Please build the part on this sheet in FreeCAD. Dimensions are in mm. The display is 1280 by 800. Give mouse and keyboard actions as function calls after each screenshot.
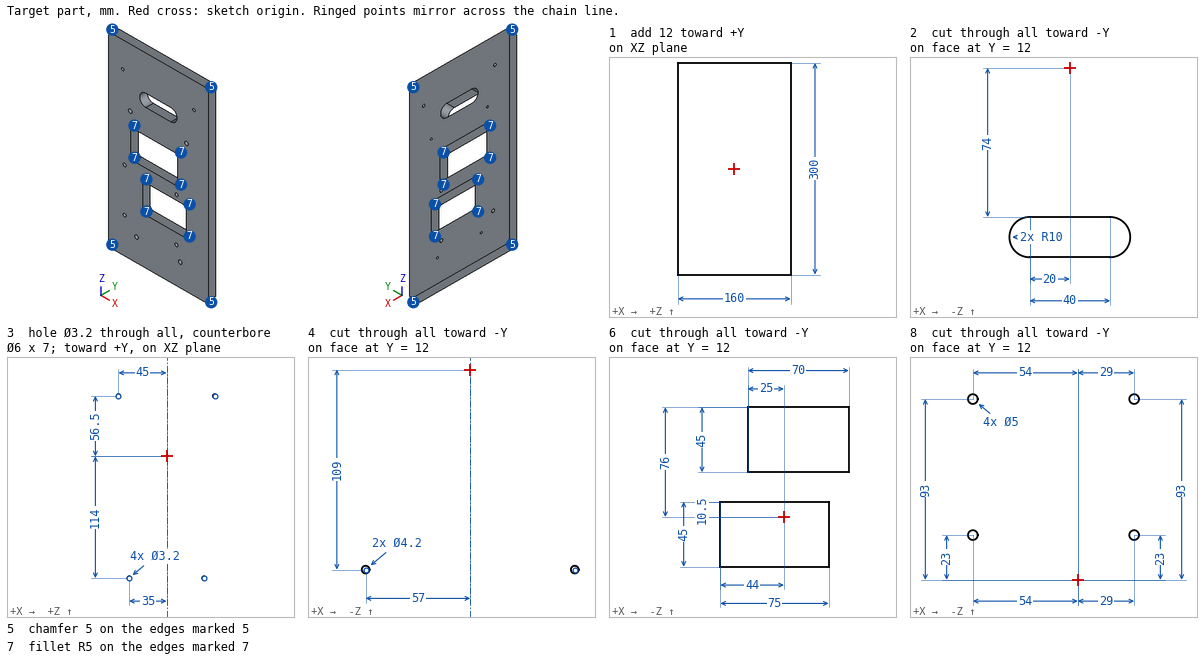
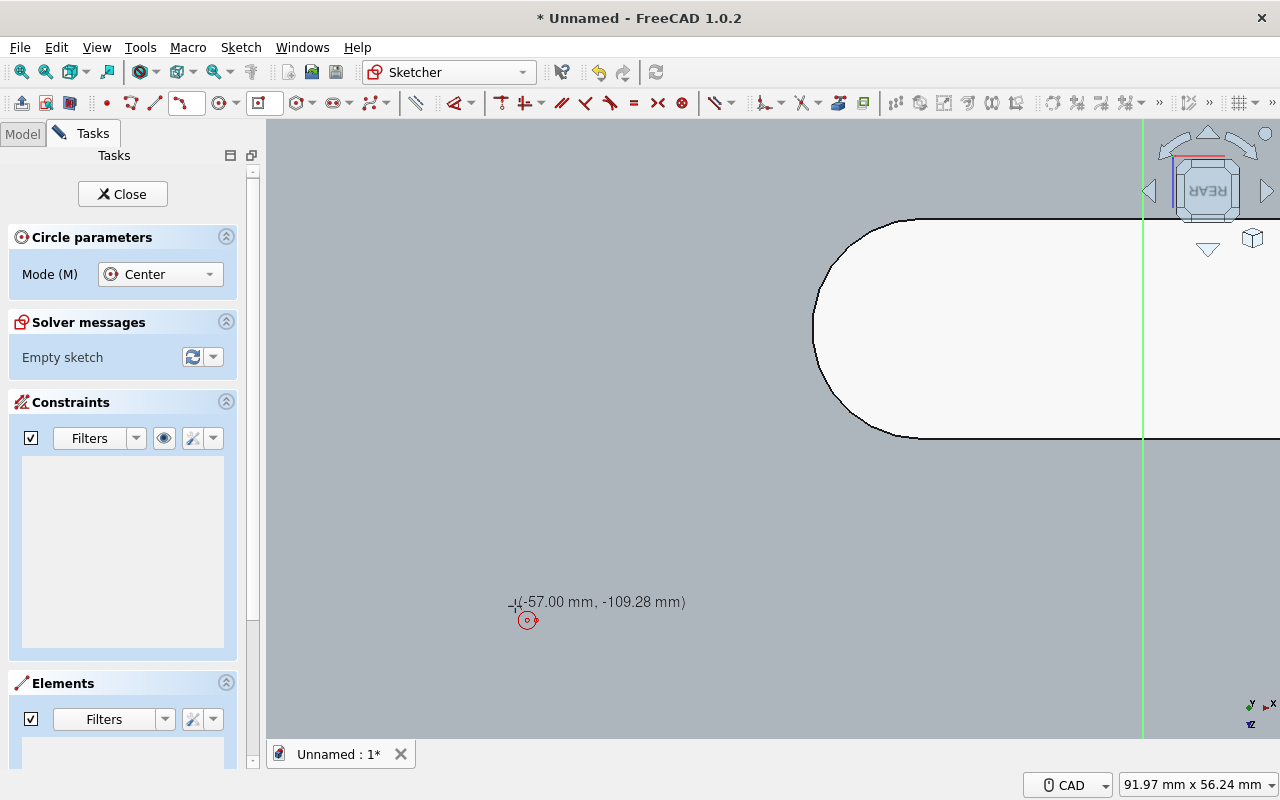
click(514, 604)
click(531, 588)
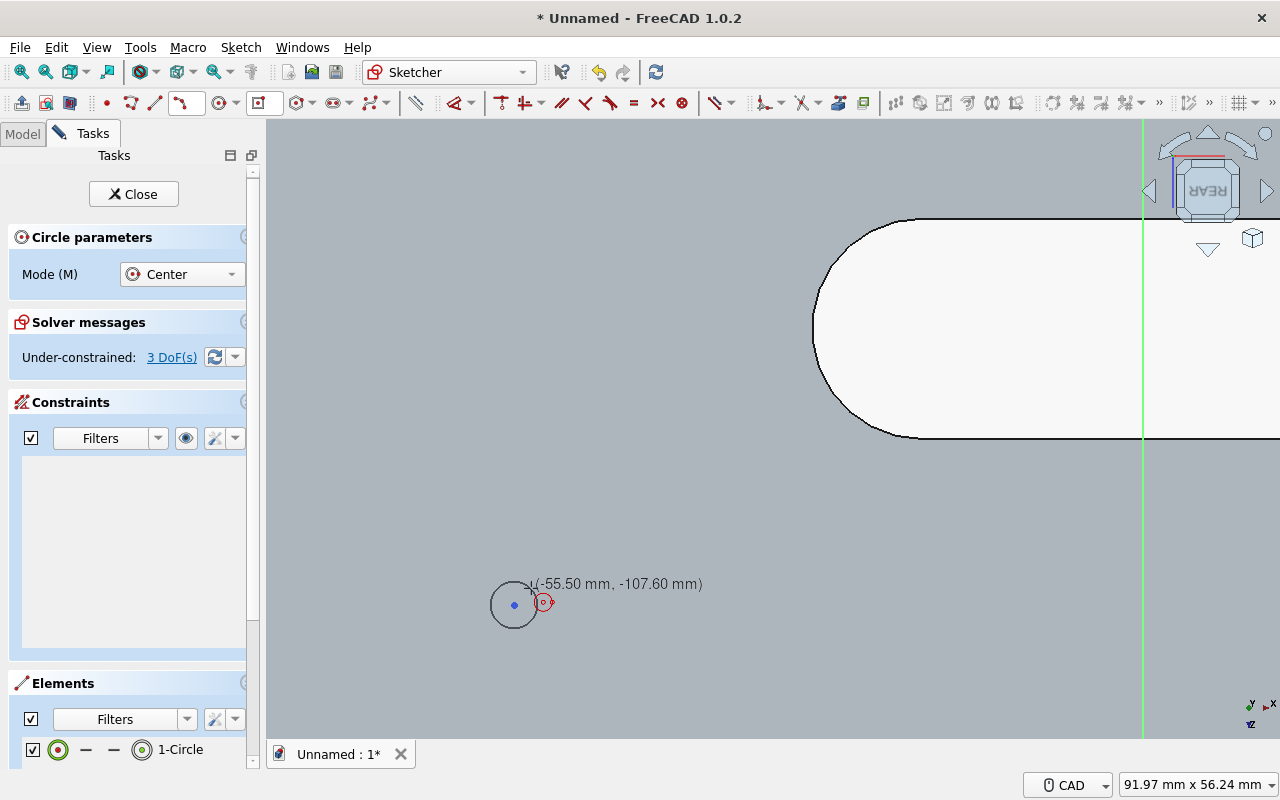
scroll(516, 607, down, 6)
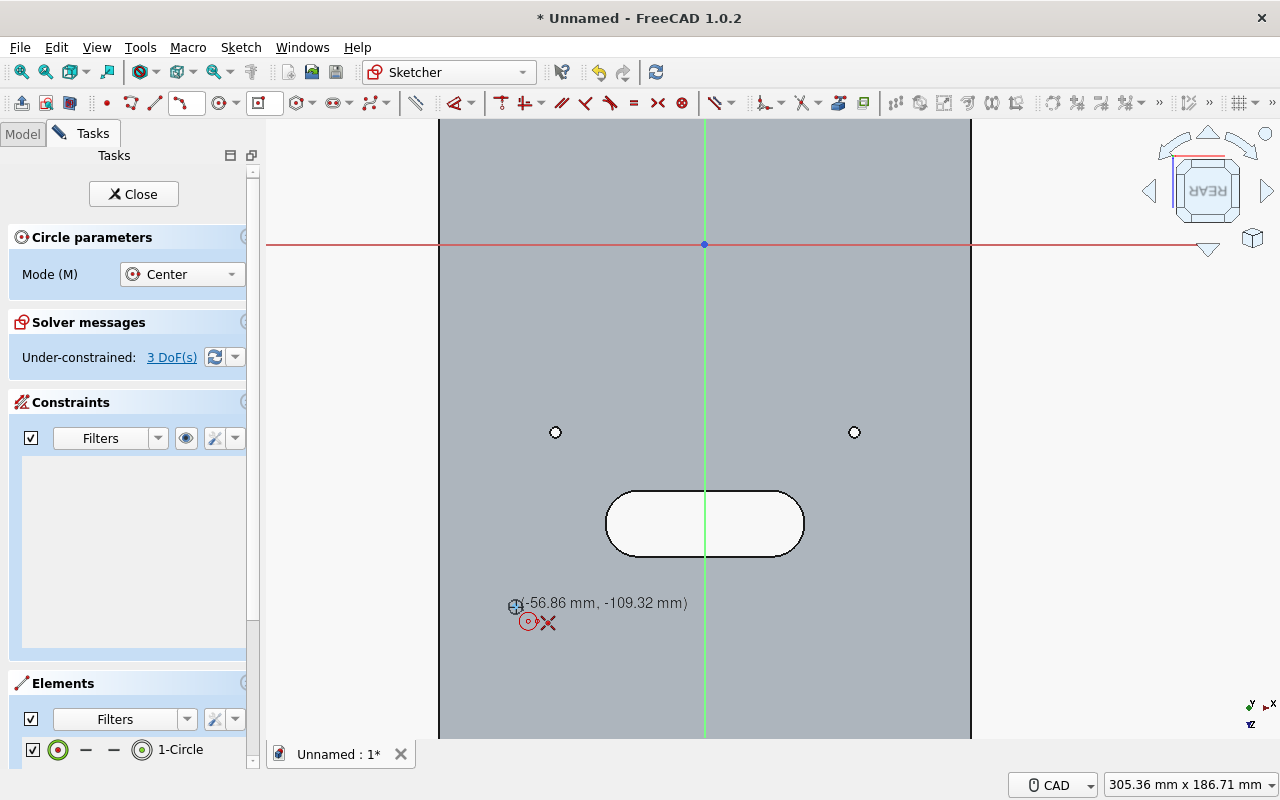
scroll(894, 607, up, 6)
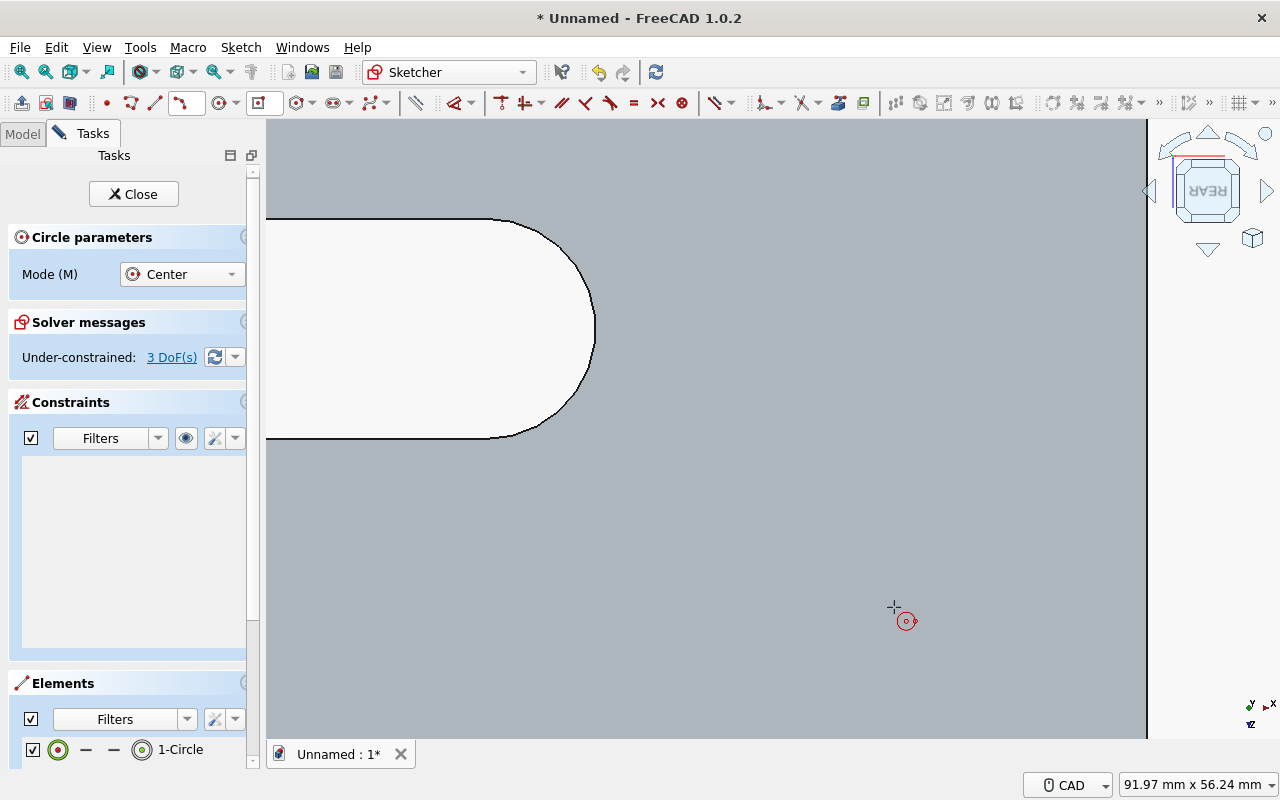
click(893, 604)
click(910, 588)
key(Escape)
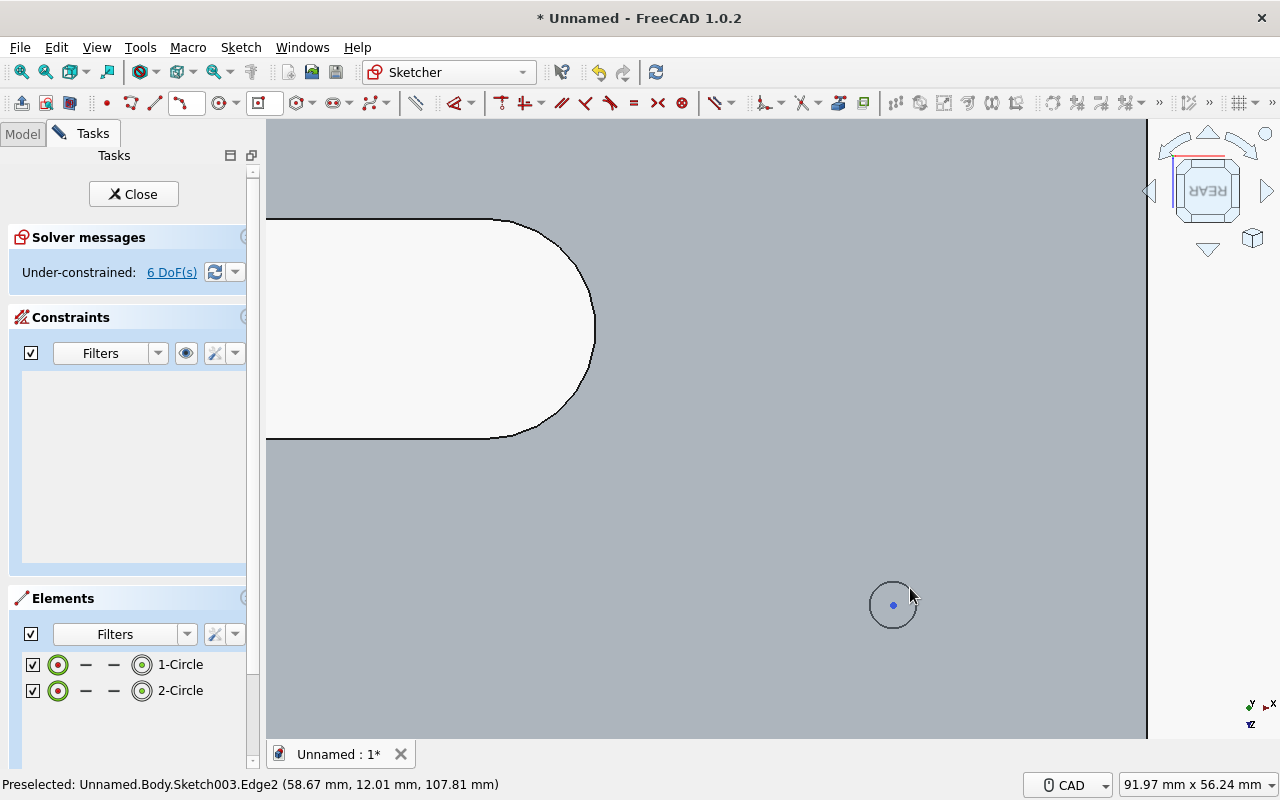
scroll(894, 607, down, 6)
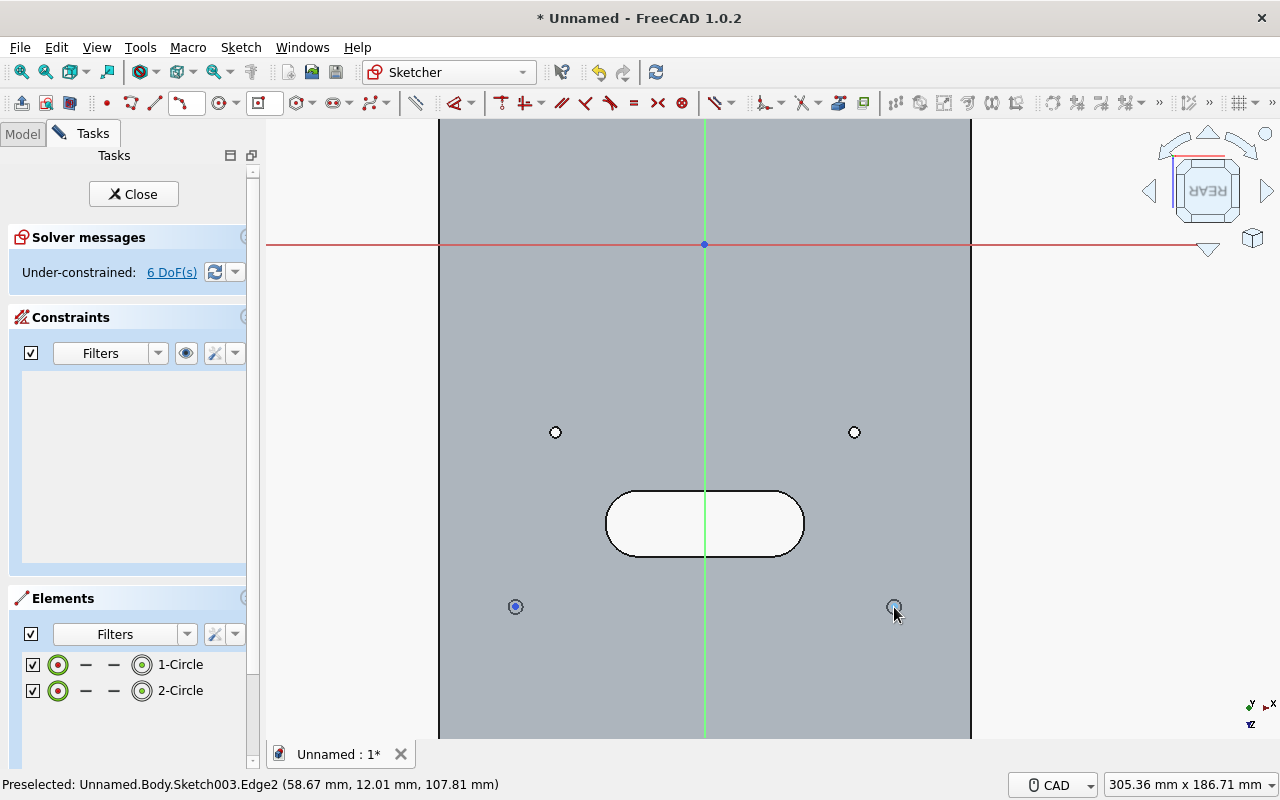
scroll(521, 602, up, 4)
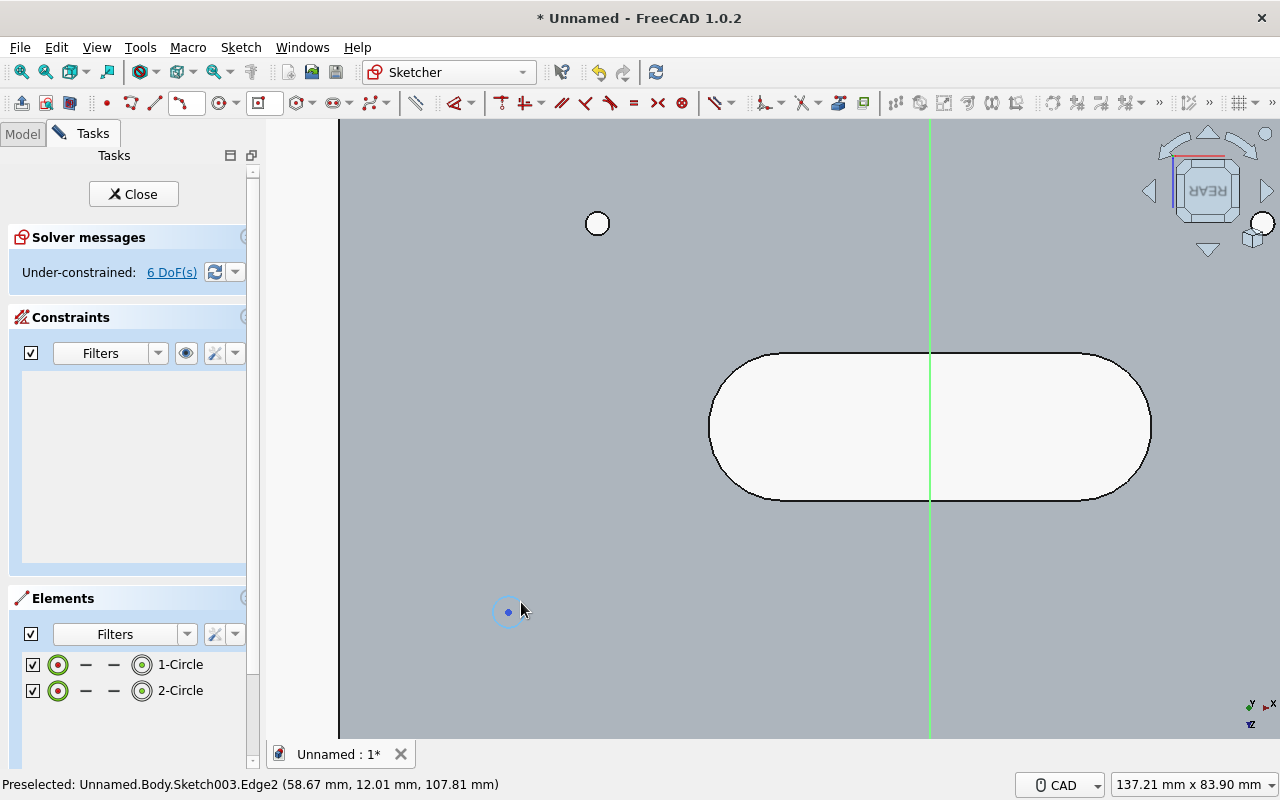
click(520, 601)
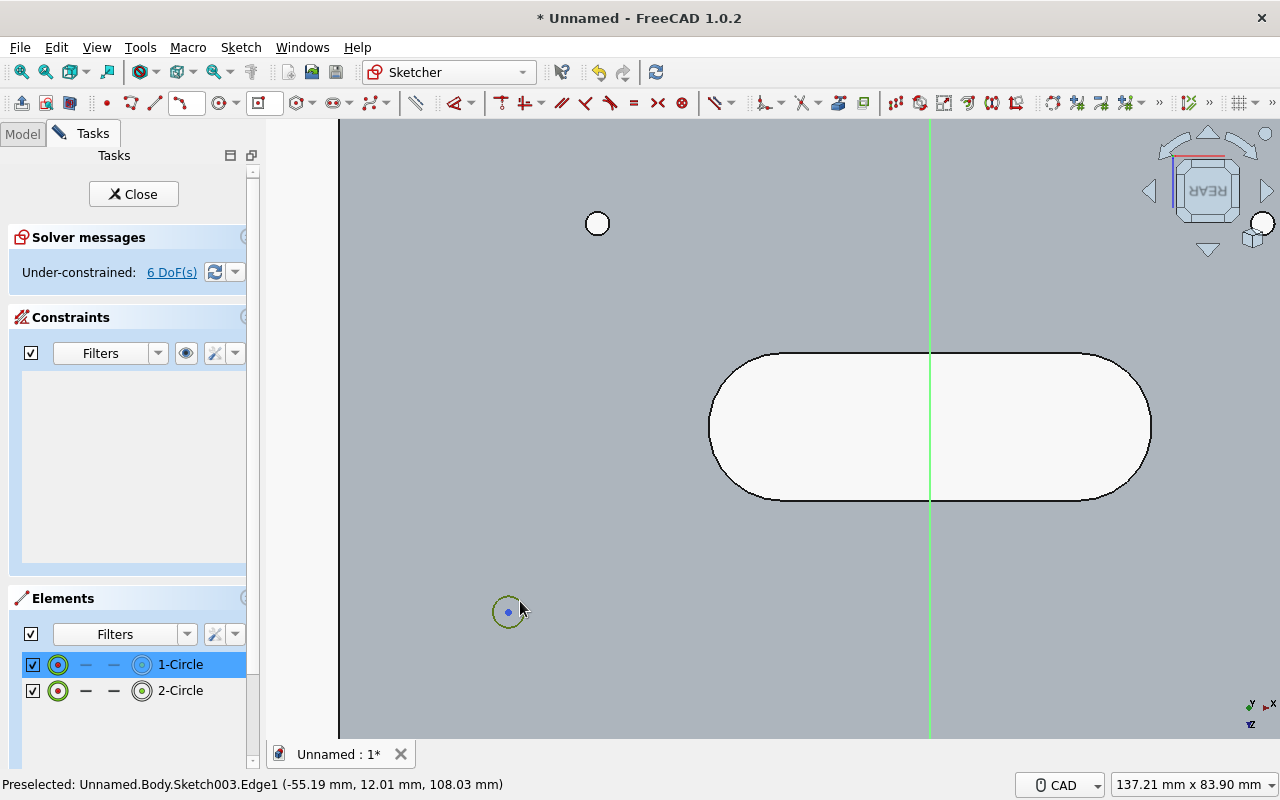
scroll(520, 602, down, 4)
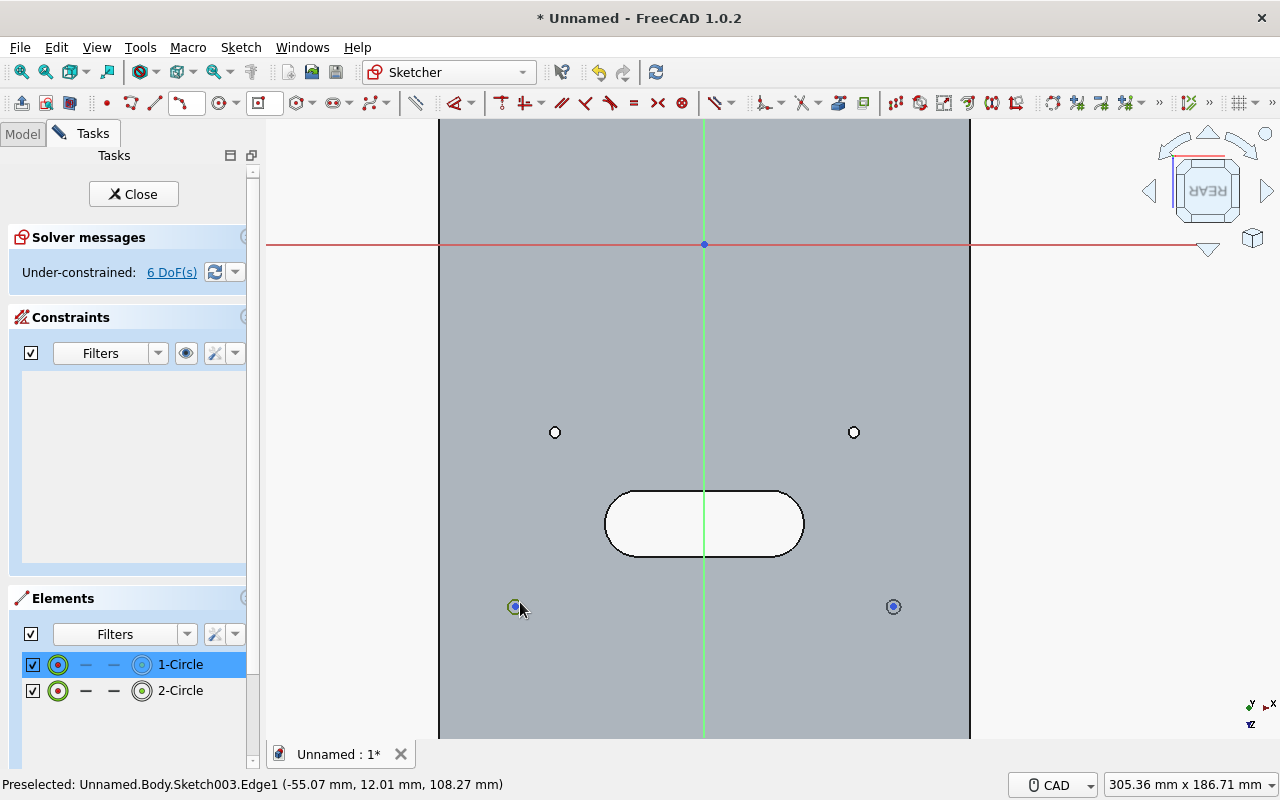
scroll(899, 602, up, 4)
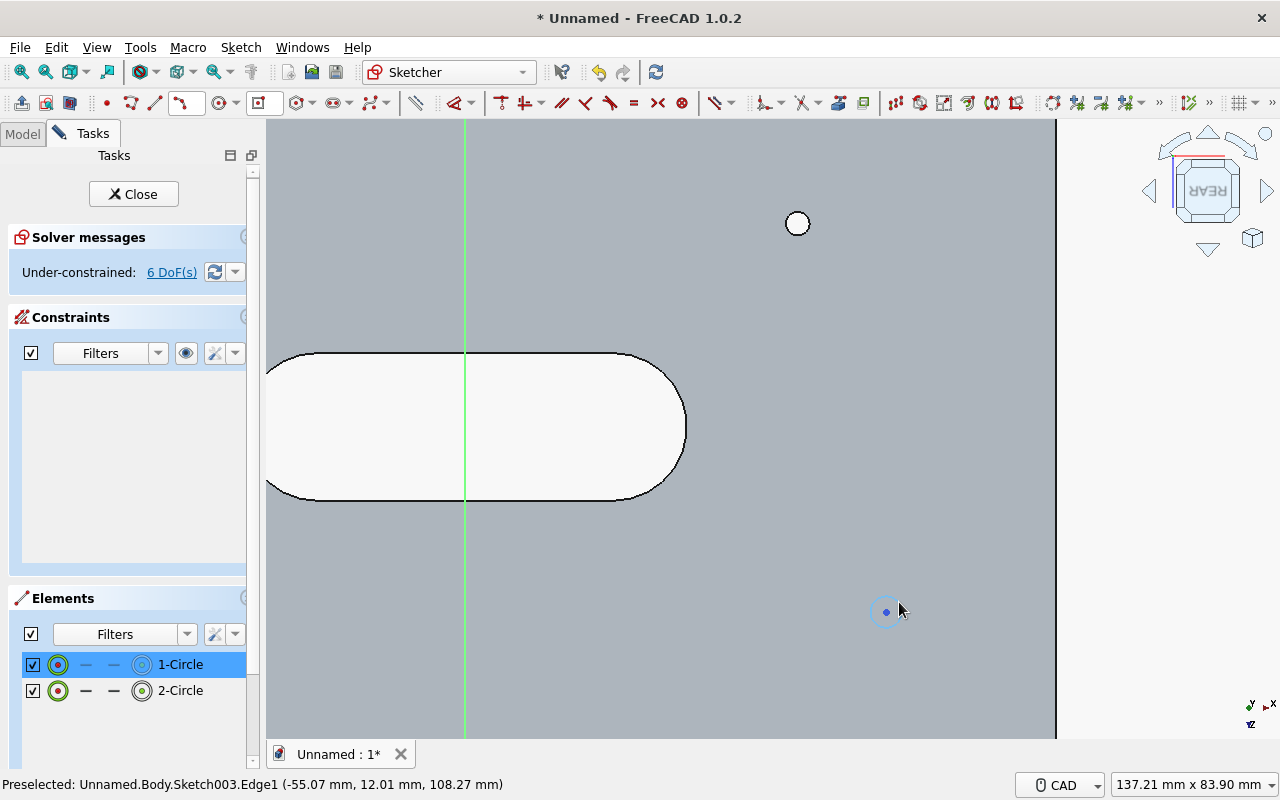
click(897, 601)